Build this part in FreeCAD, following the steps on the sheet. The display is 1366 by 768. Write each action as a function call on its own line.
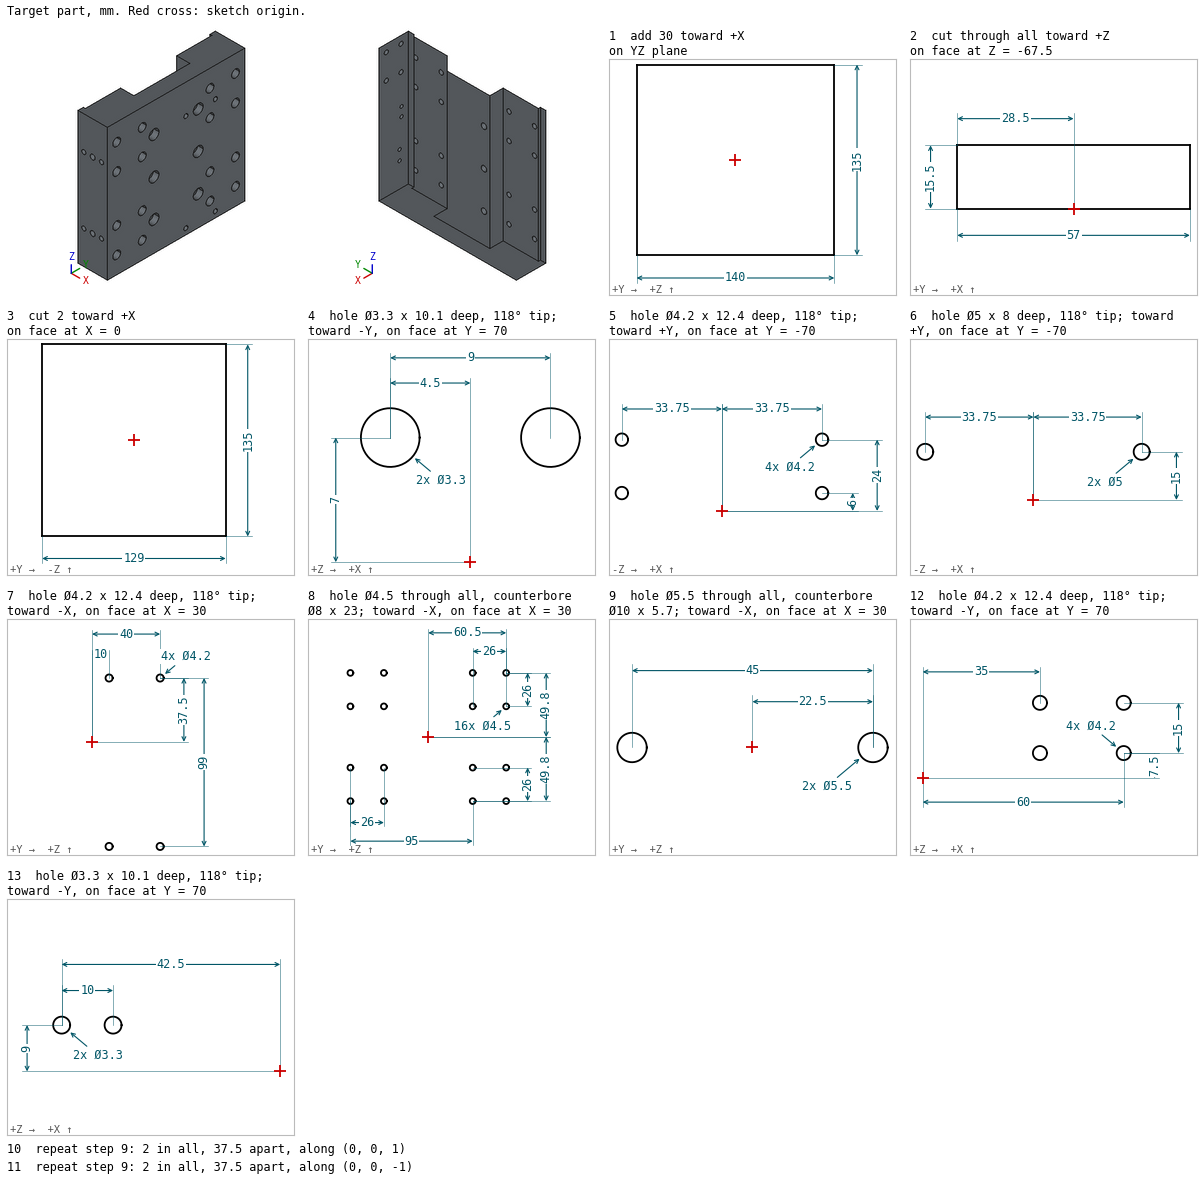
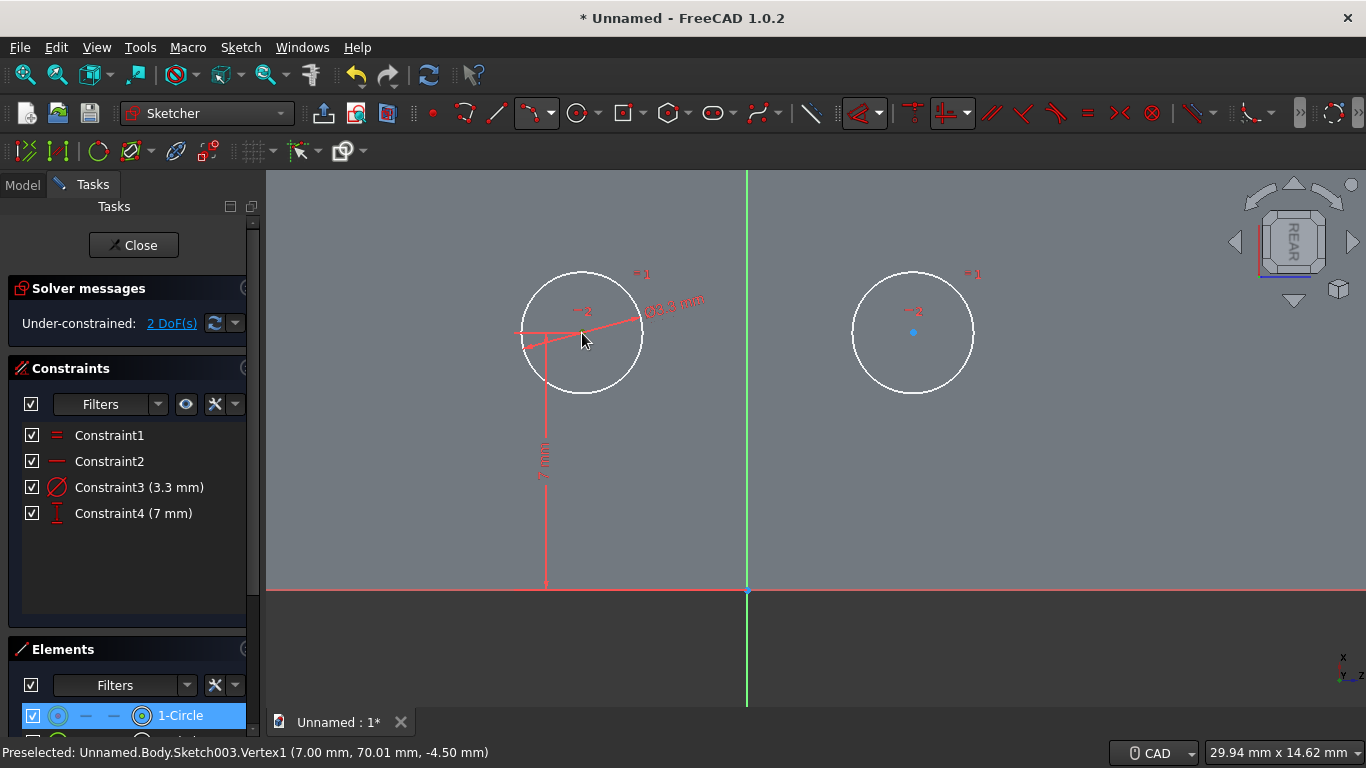
click(913, 333)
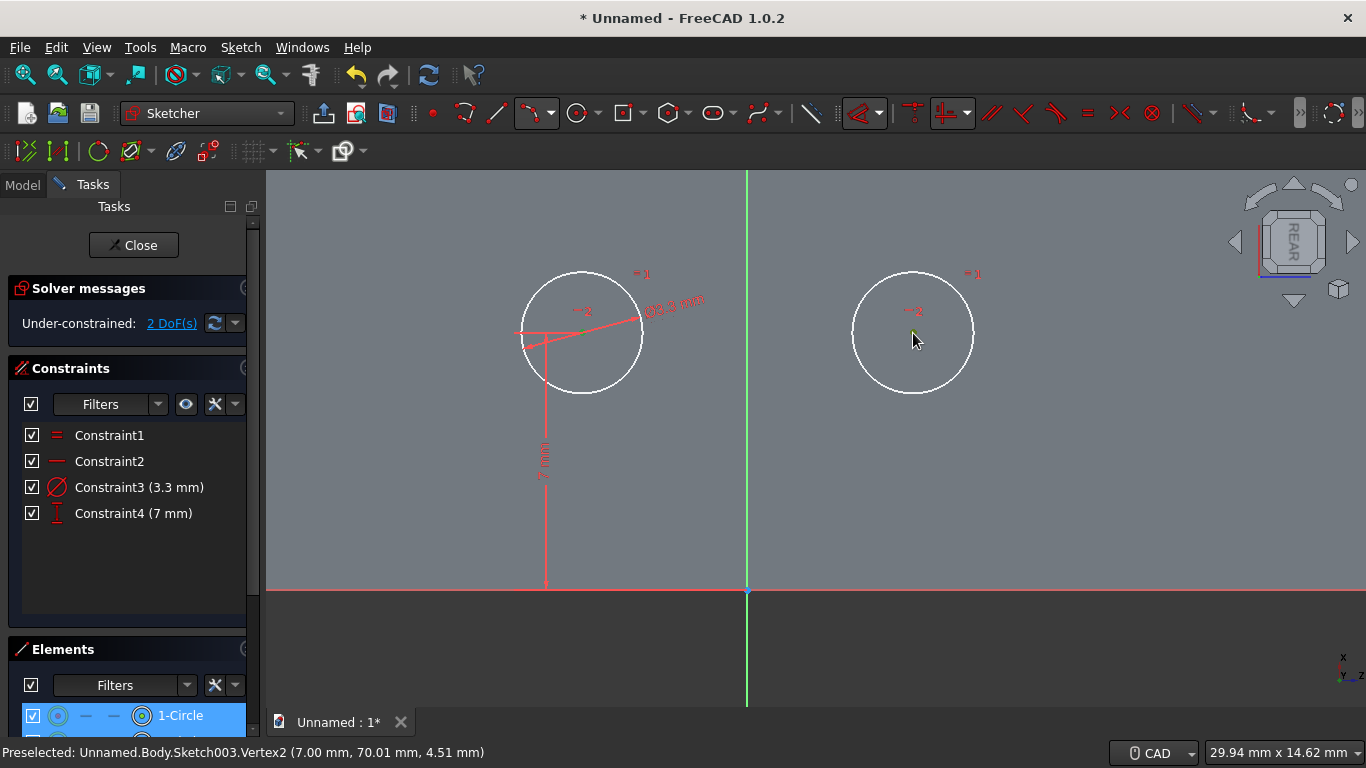
click(882, 114)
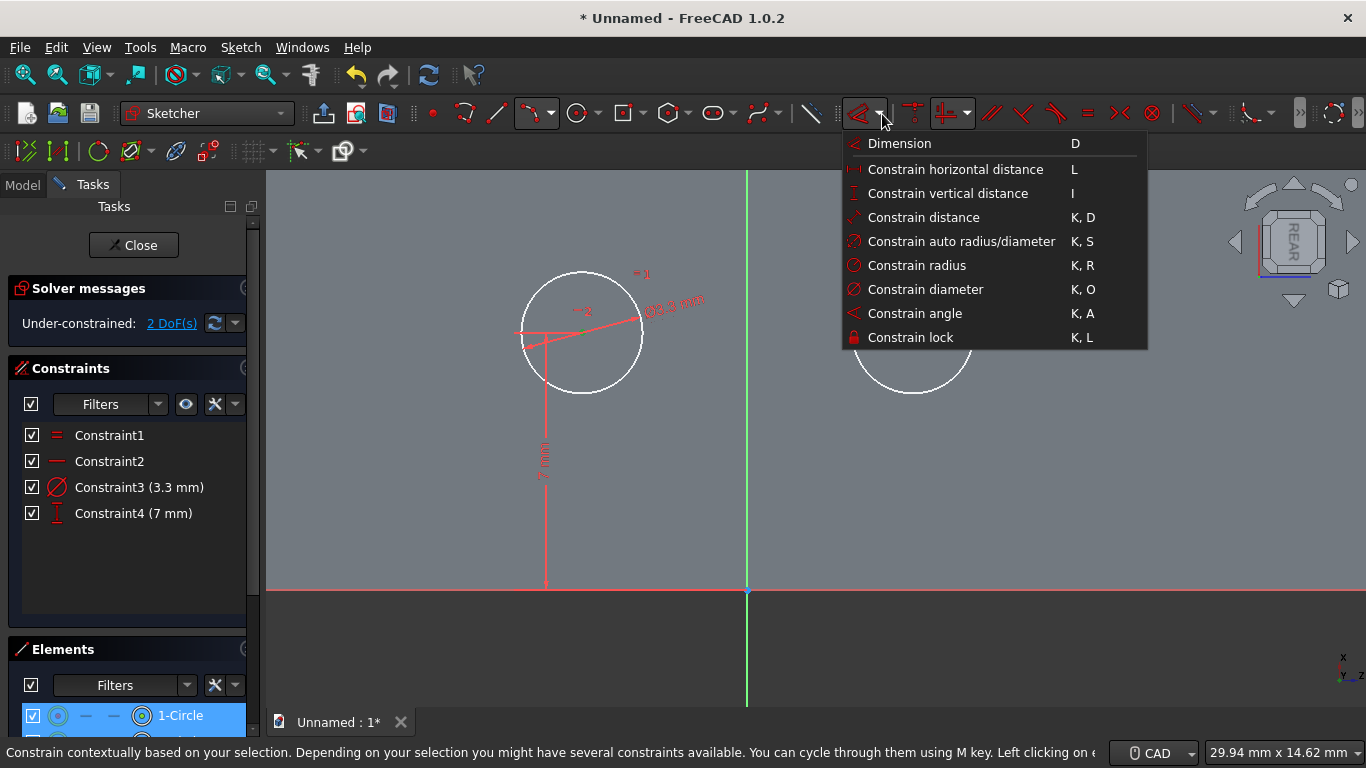
click(995, 169)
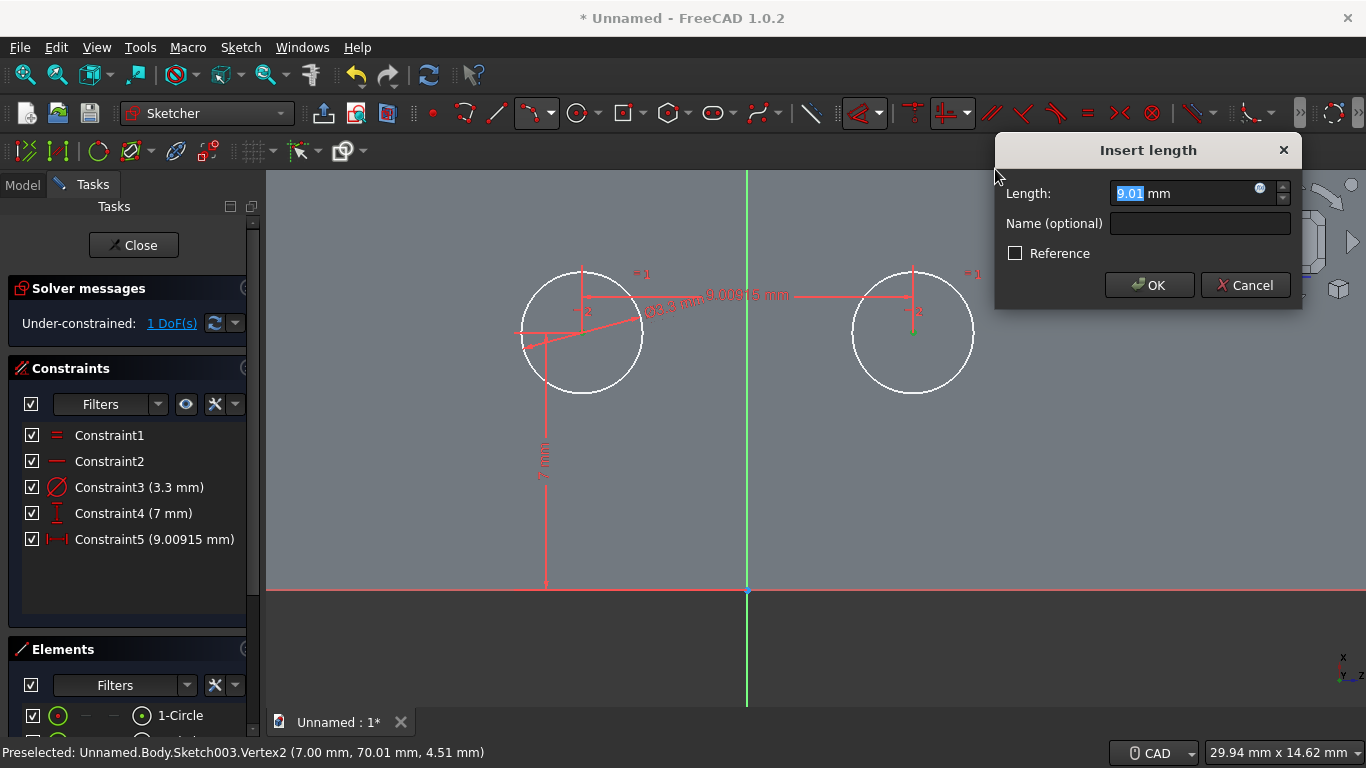
text(9)
key(Return)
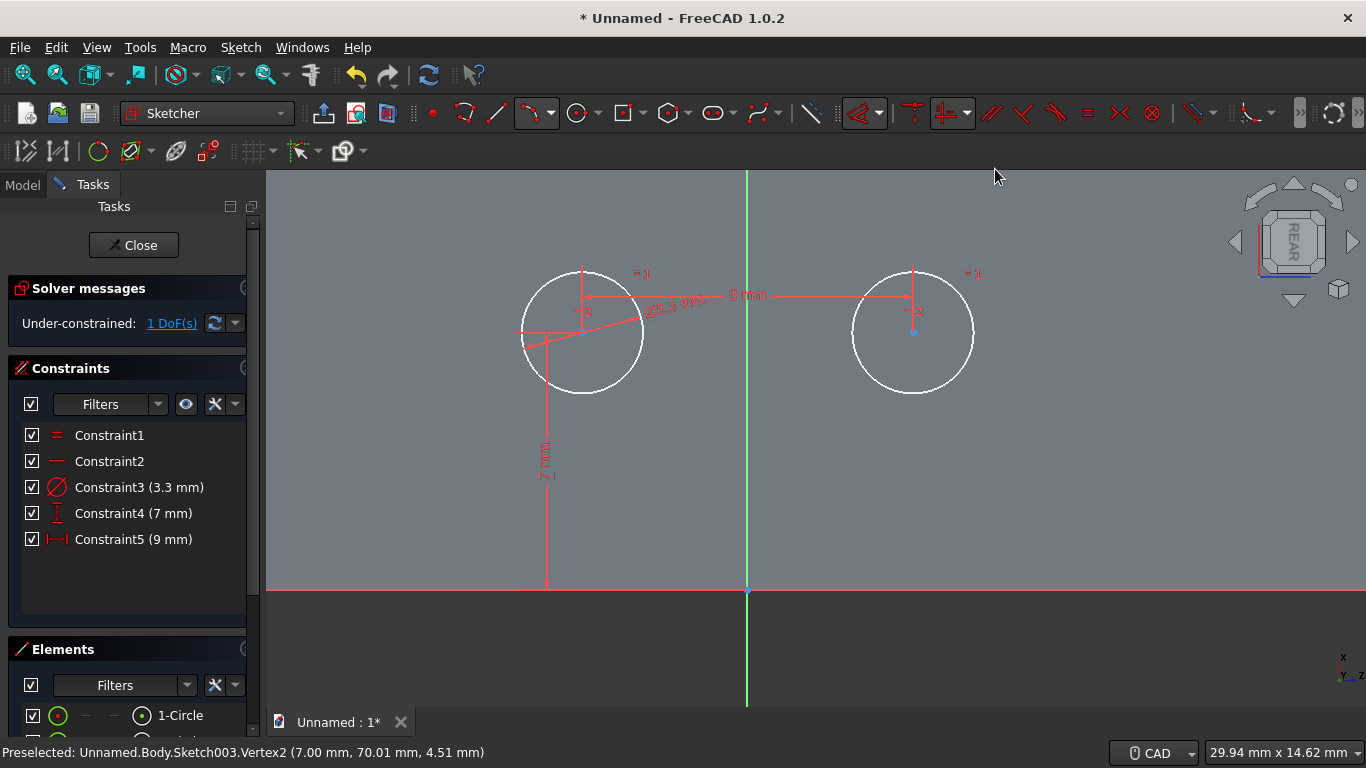
click(582, 333)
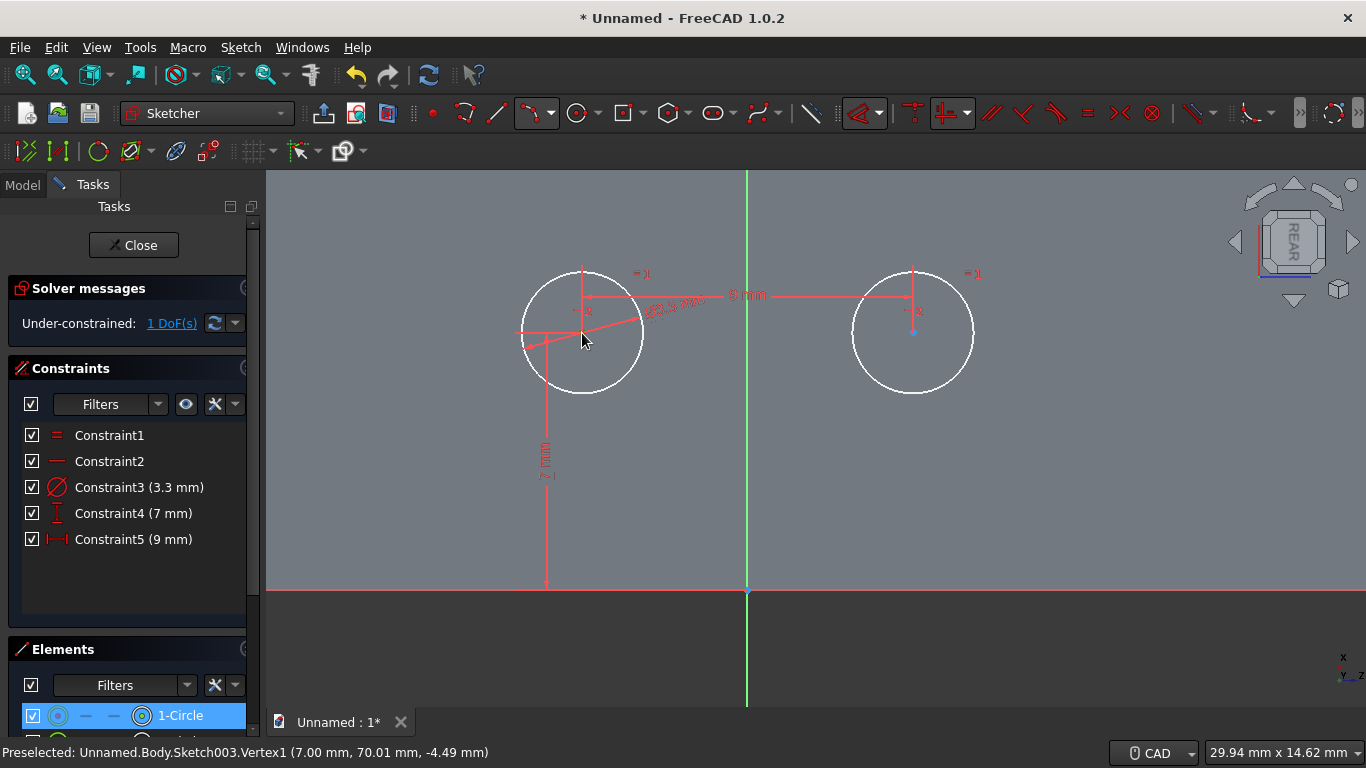
click(882, 114)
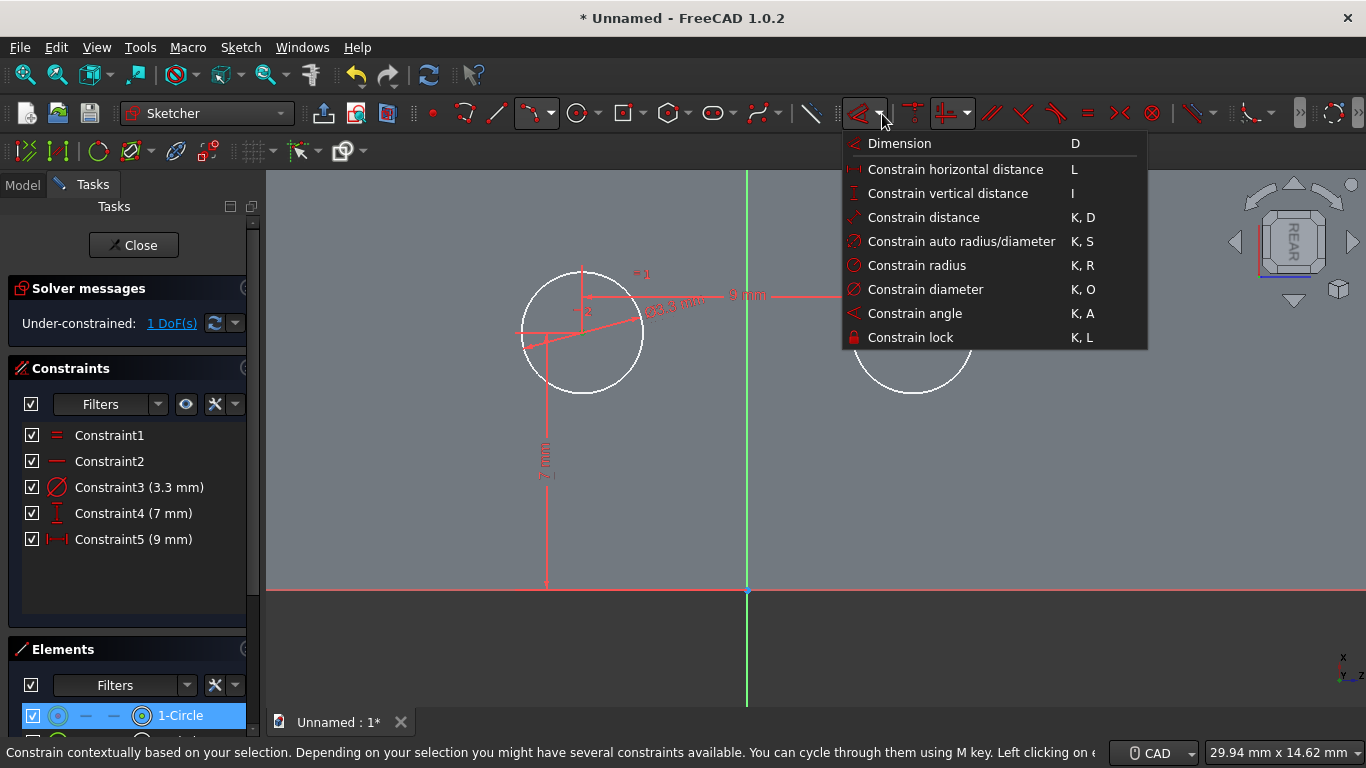
click(995, 169)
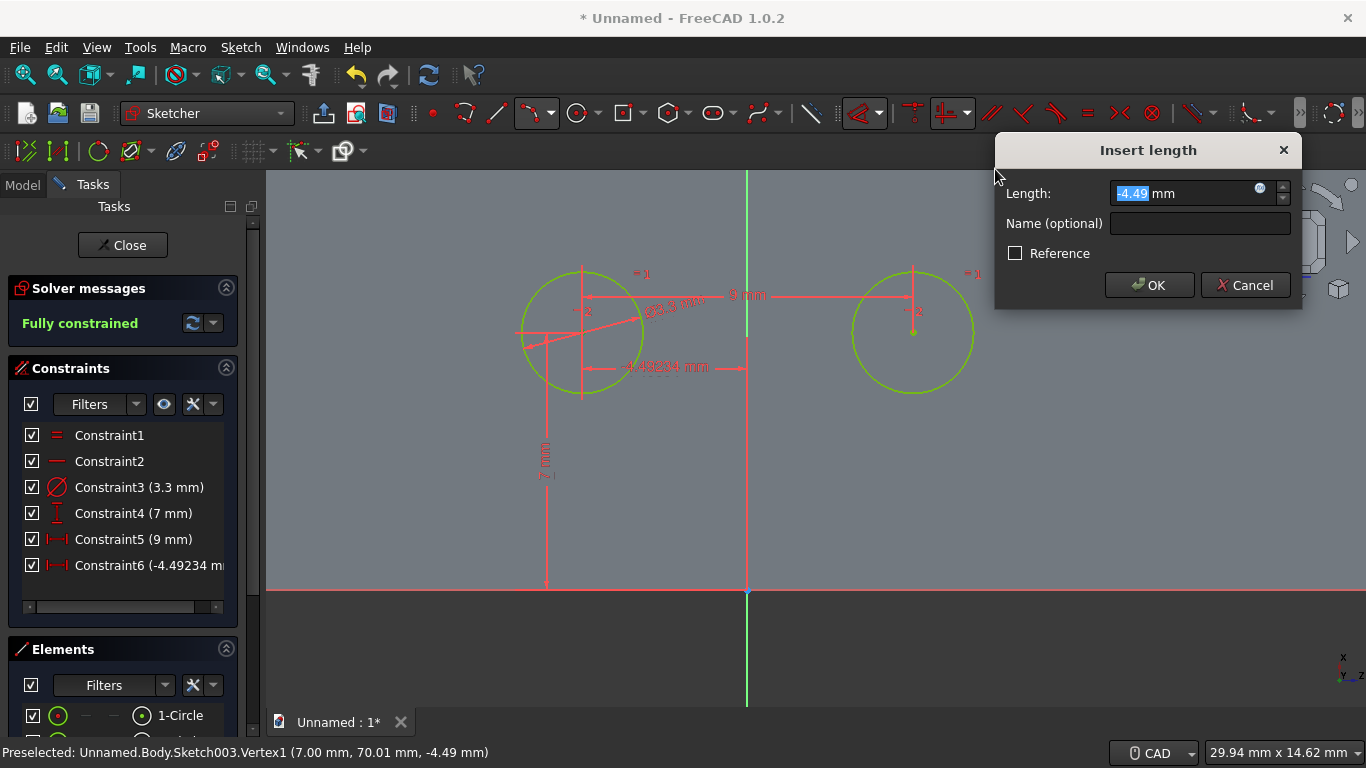
text(-4.5)
key(Return)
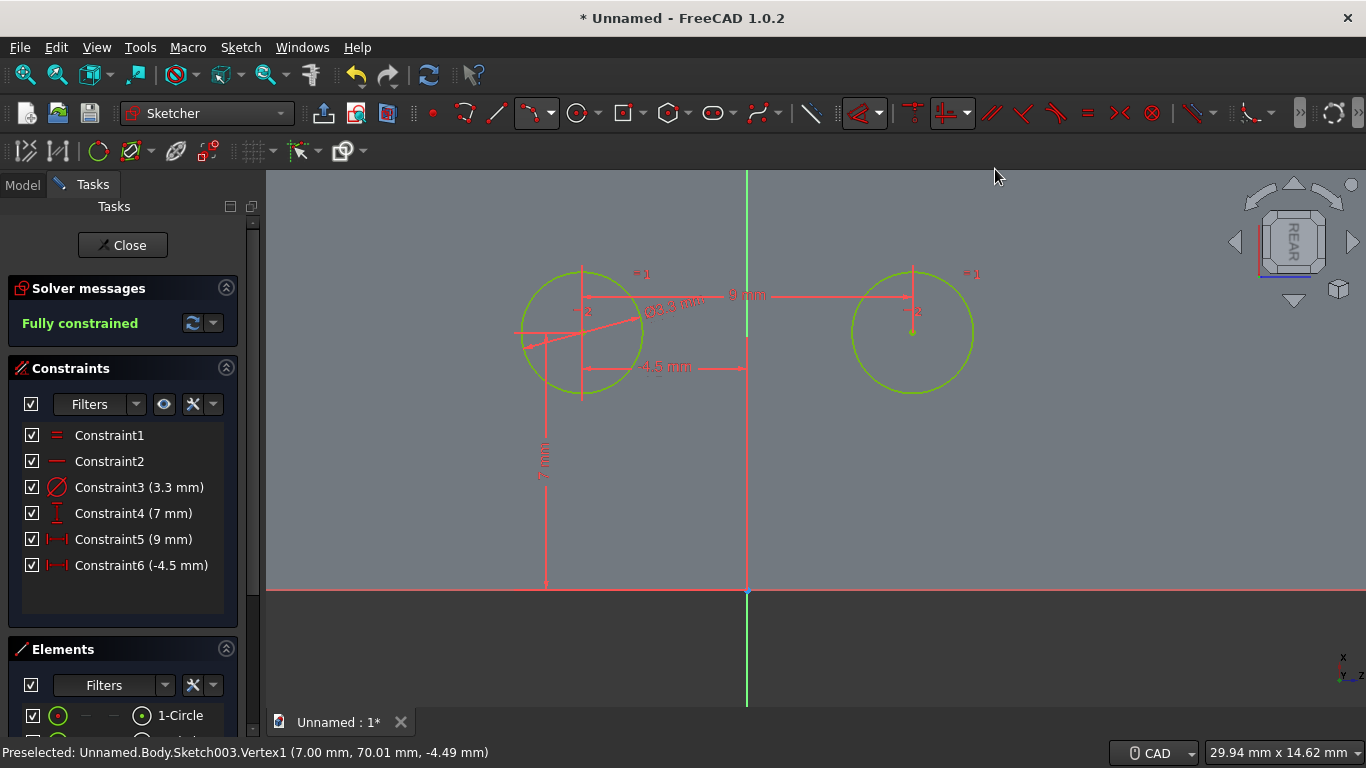
click(123, 245)